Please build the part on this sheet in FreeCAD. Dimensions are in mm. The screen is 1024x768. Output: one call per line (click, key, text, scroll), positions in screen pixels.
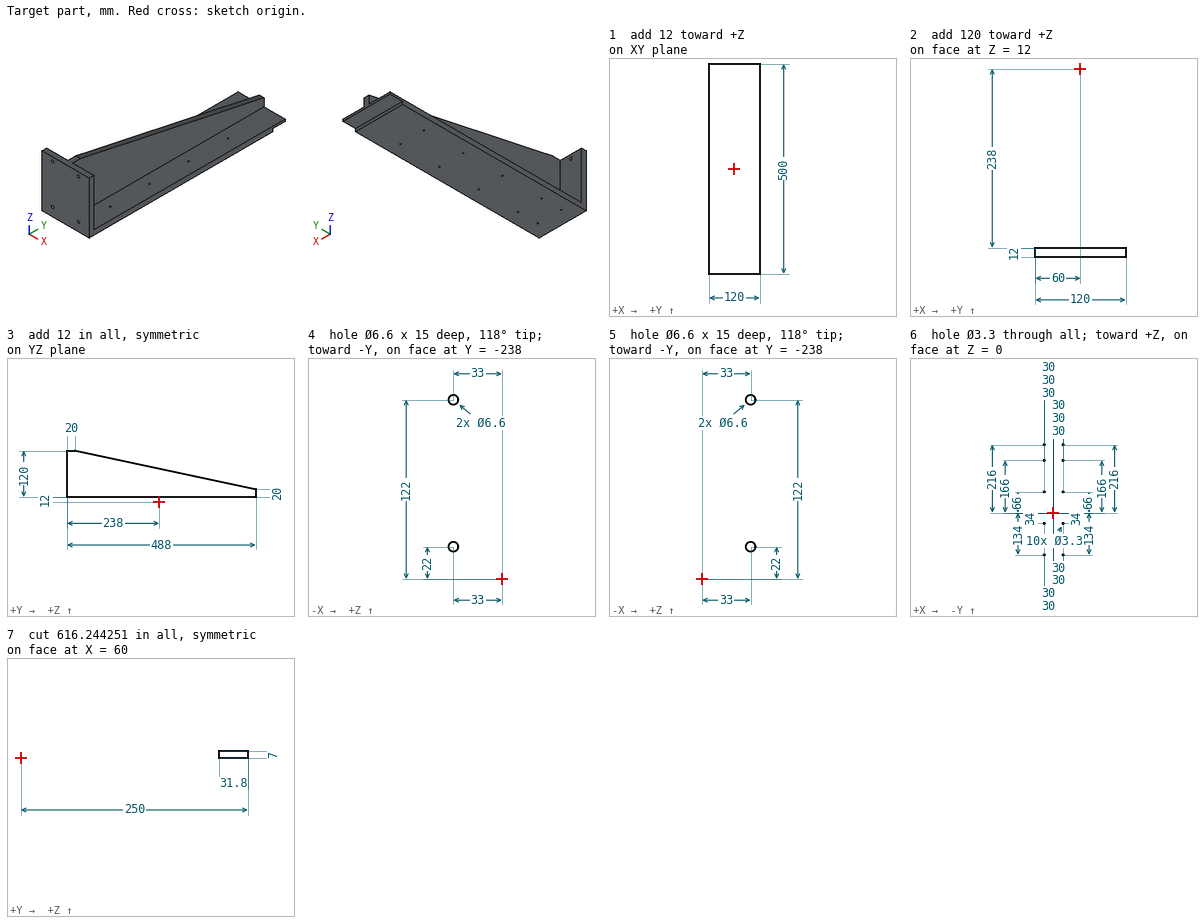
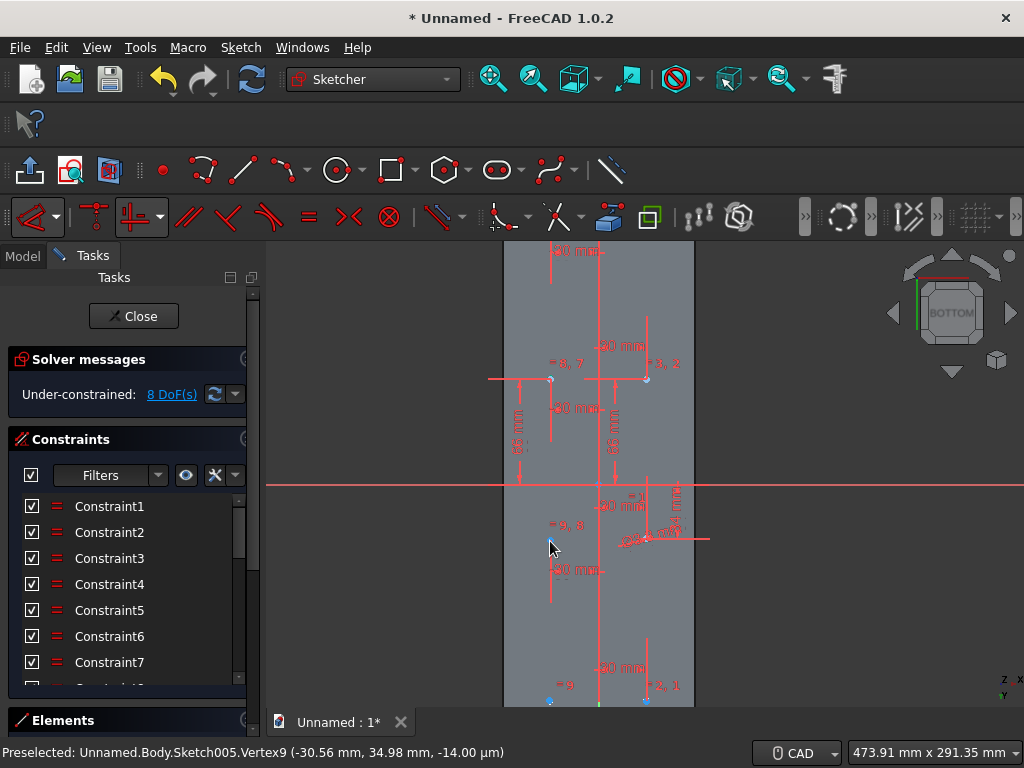
click(551, 541)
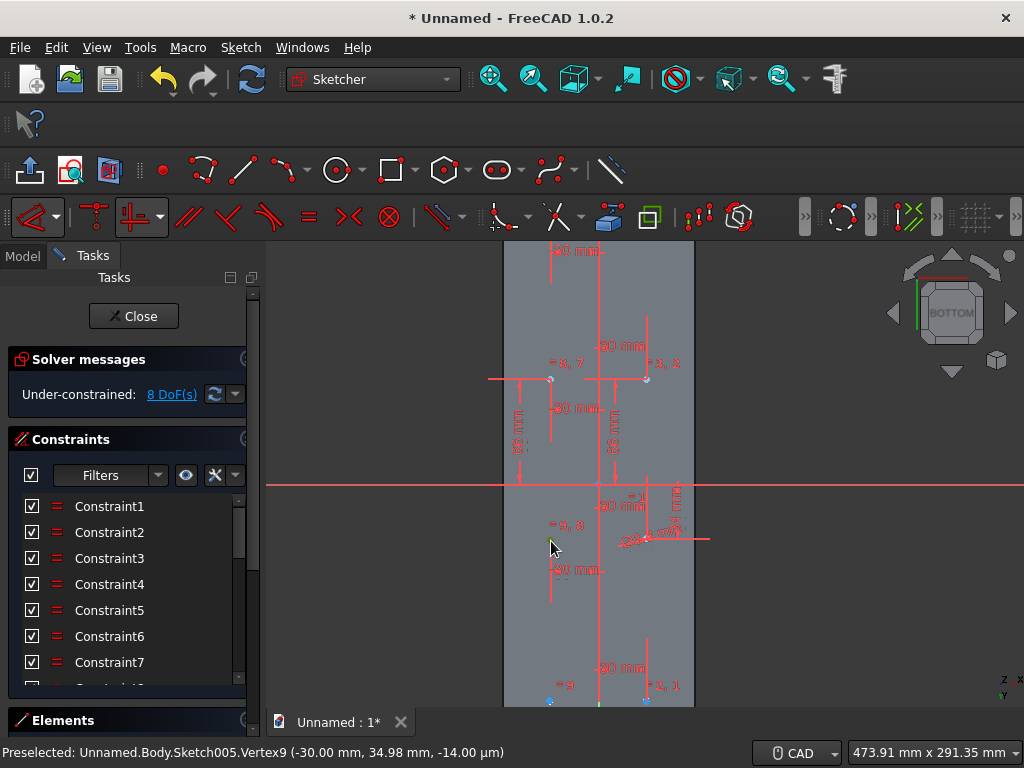
click(58, 218)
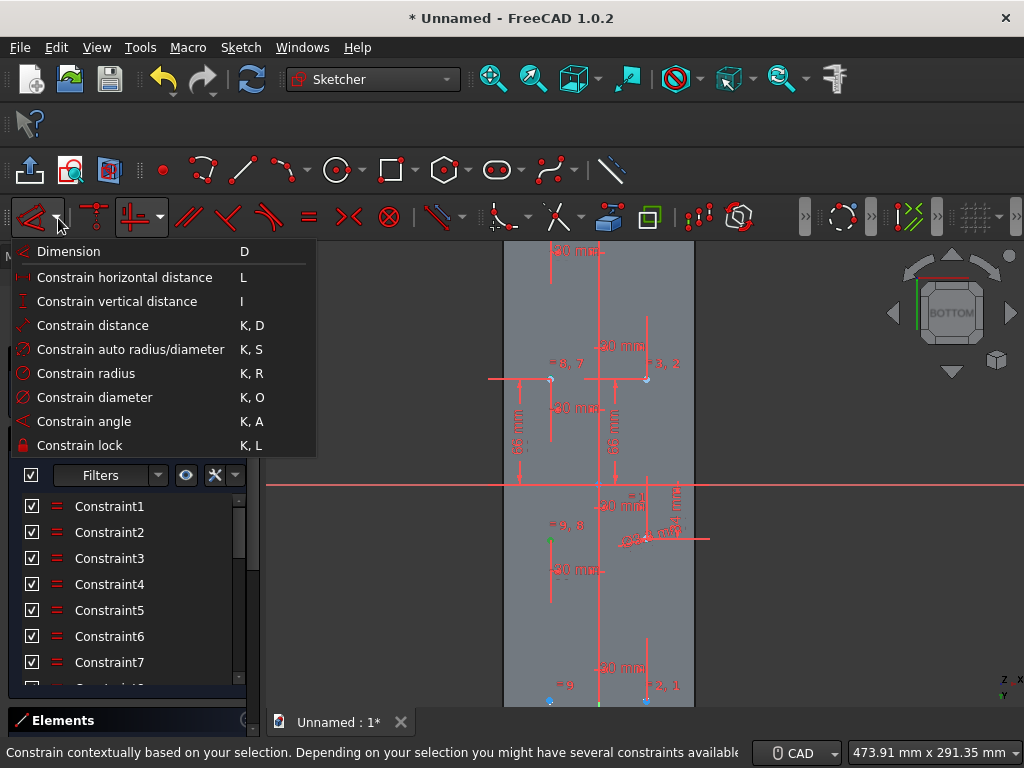
click(164, 301)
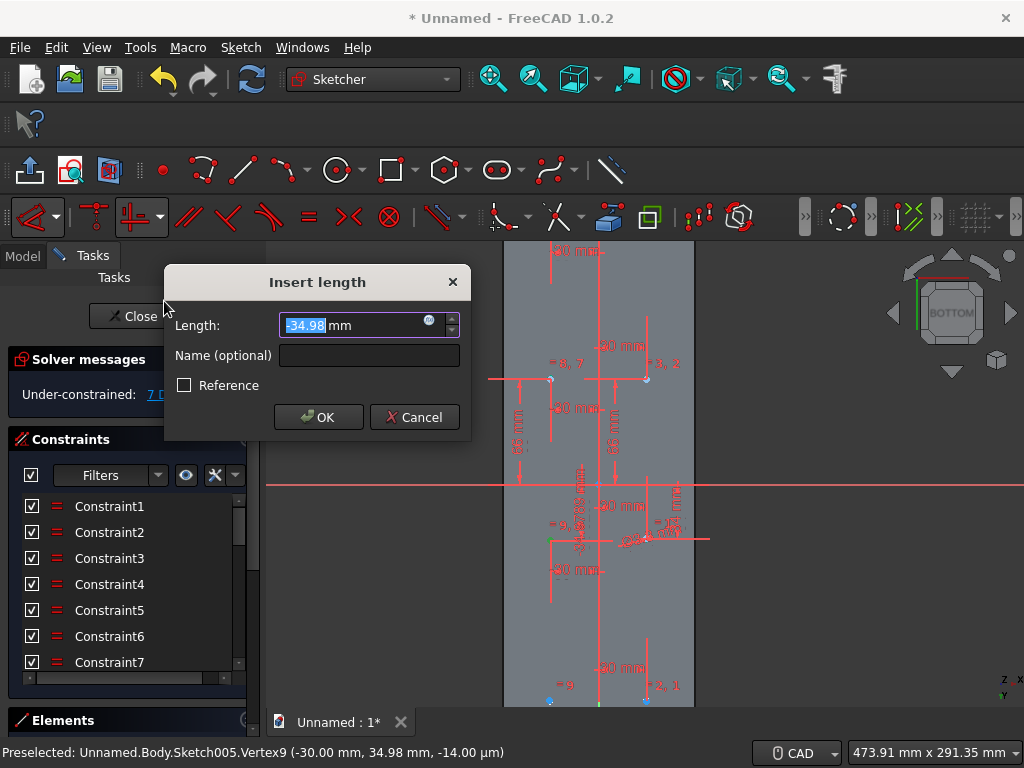
text(-34)
key(Return)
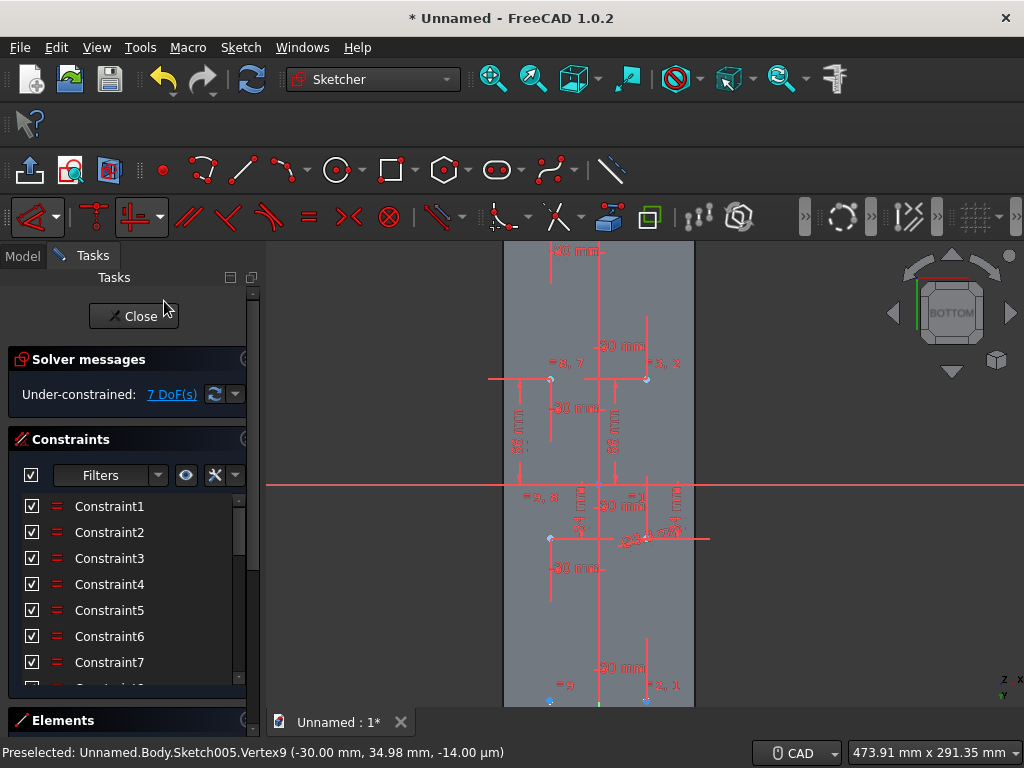
scroll(550, 541, down, 3)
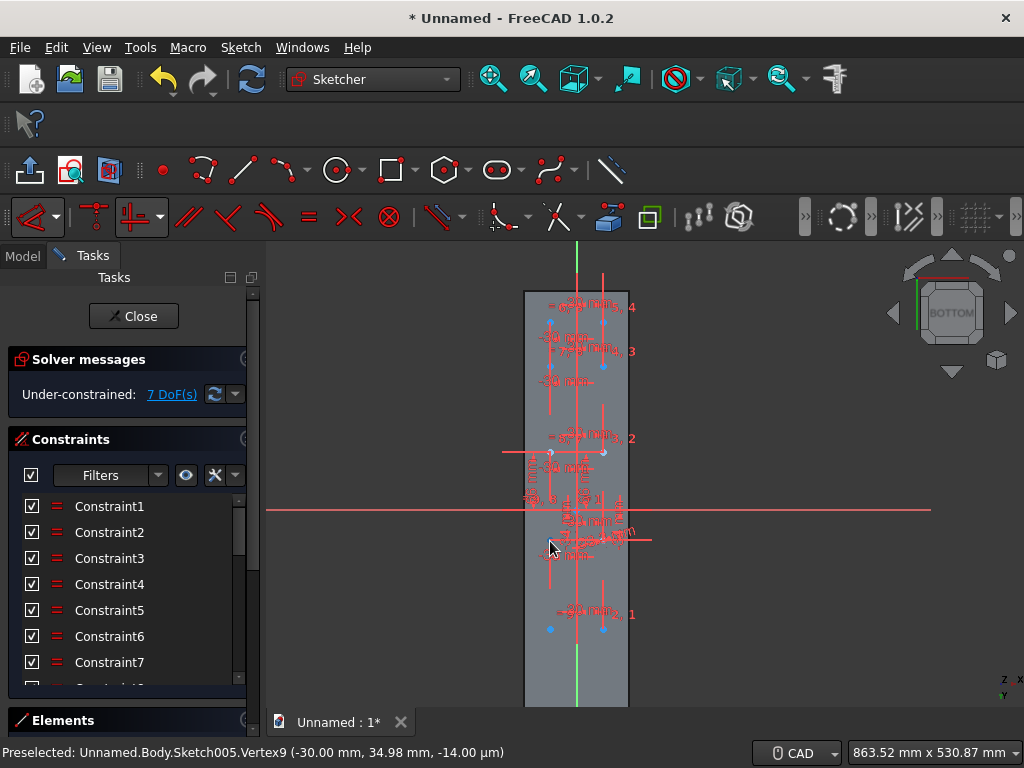
scroll(550, 629, up, 3)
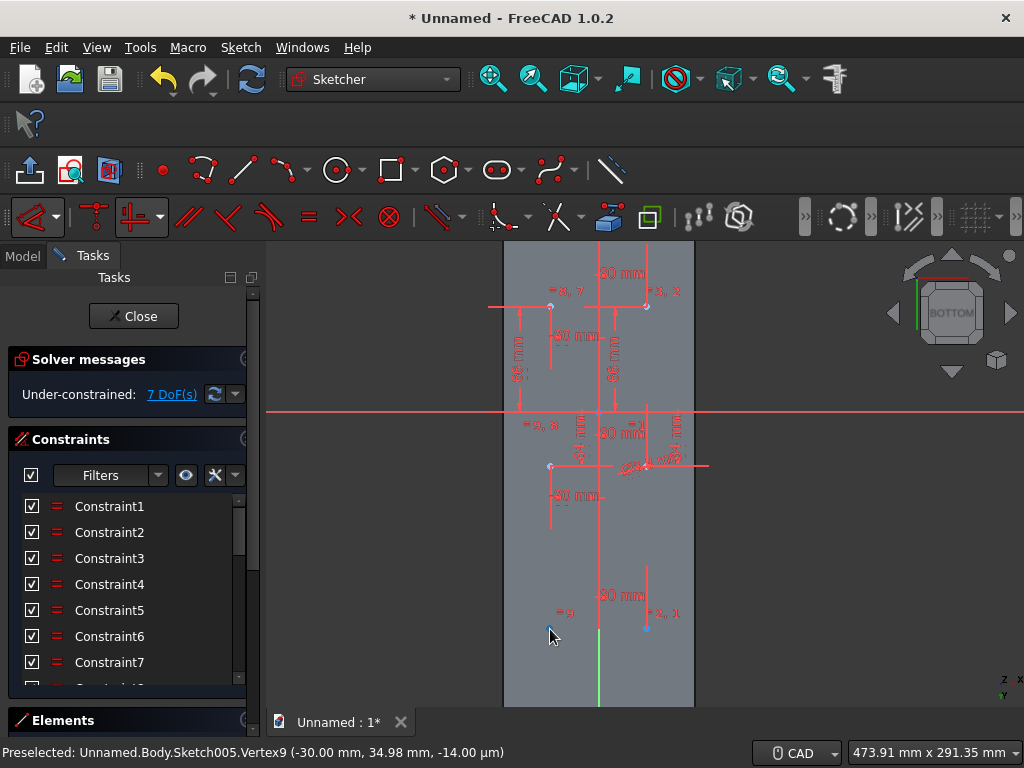
click(550, 628)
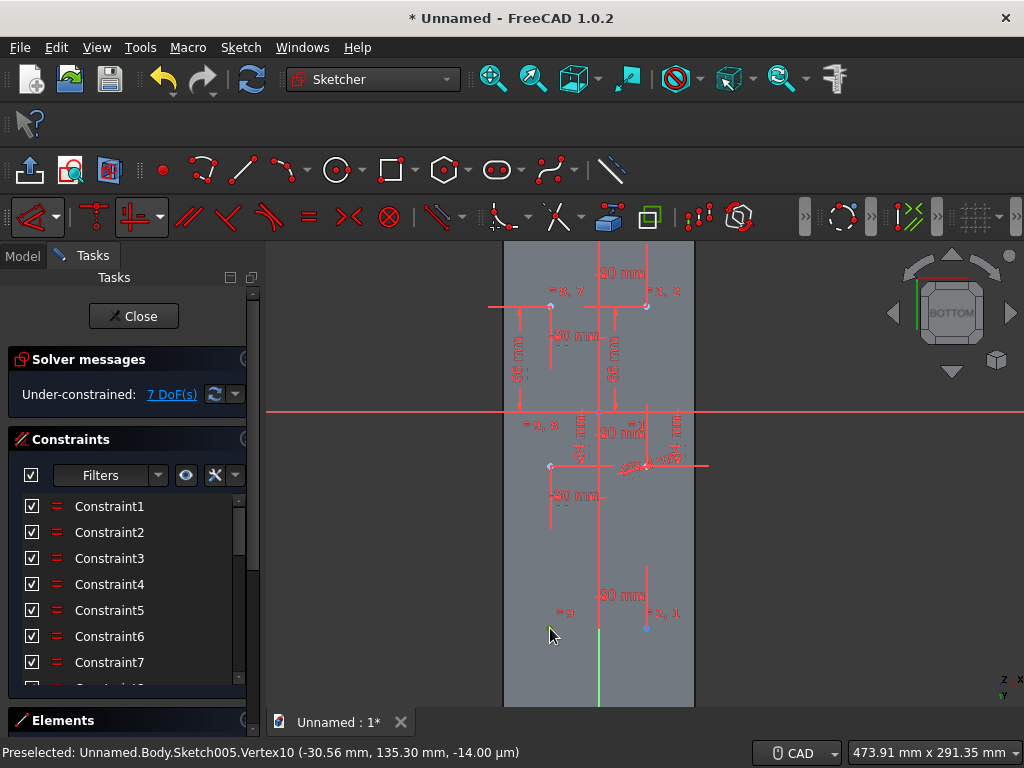
click(58, 218)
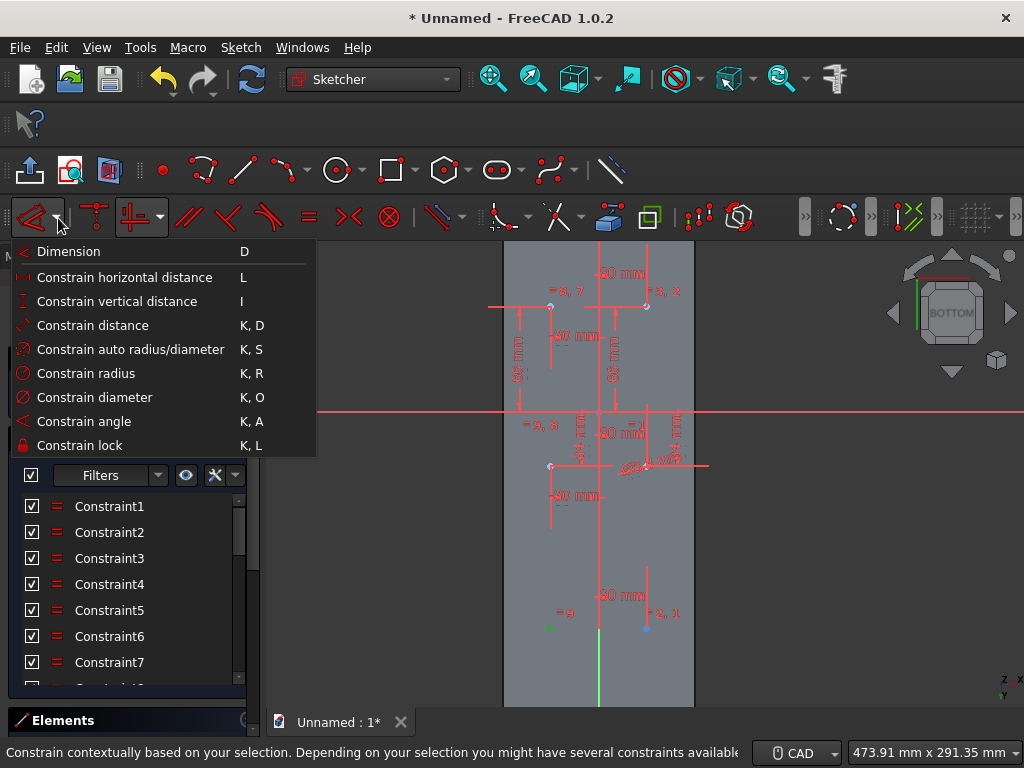
click(164, 277)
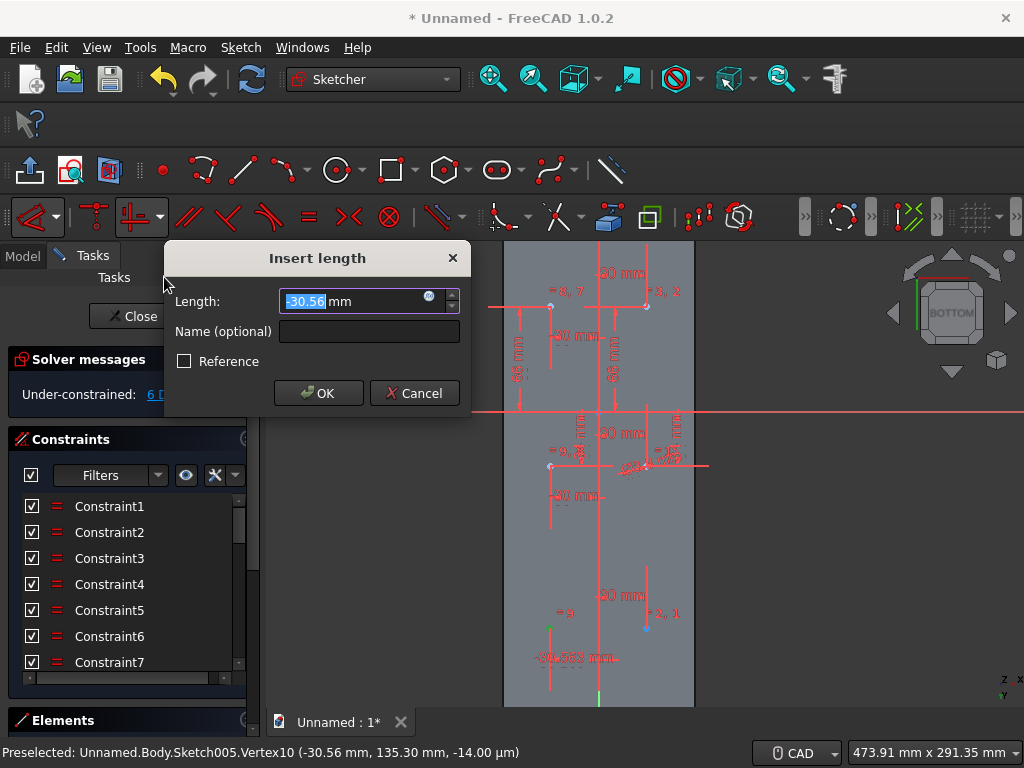
text(-30)
key(Return)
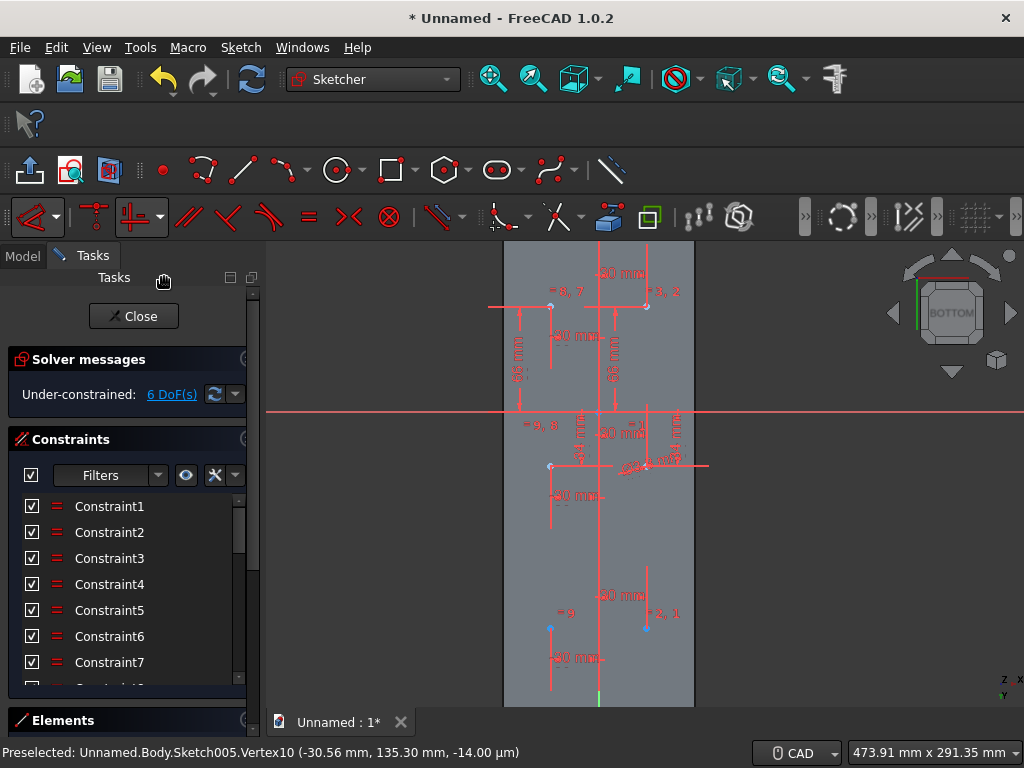
click(647, 629)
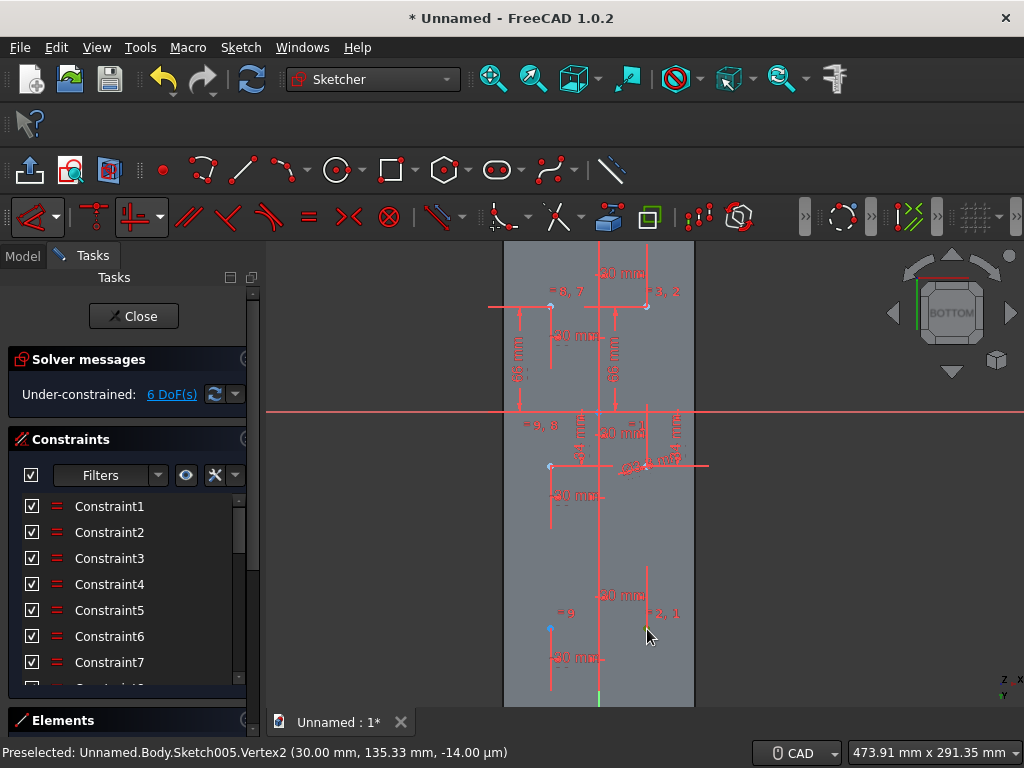
key(i)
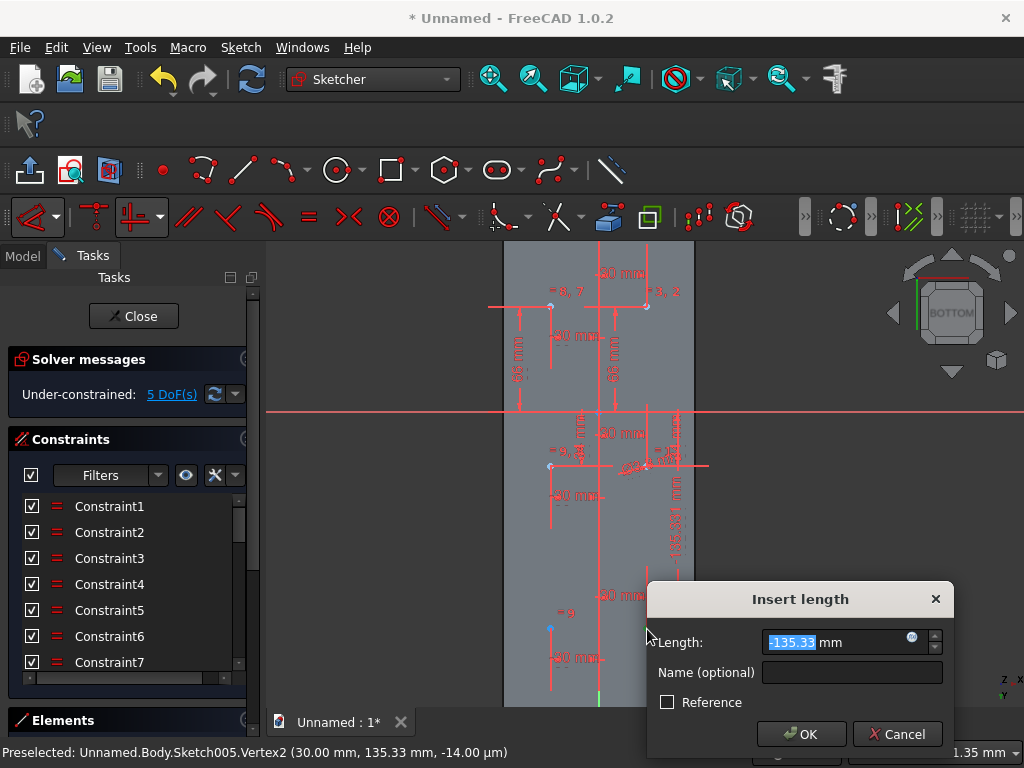
text(-134)
key(Return)